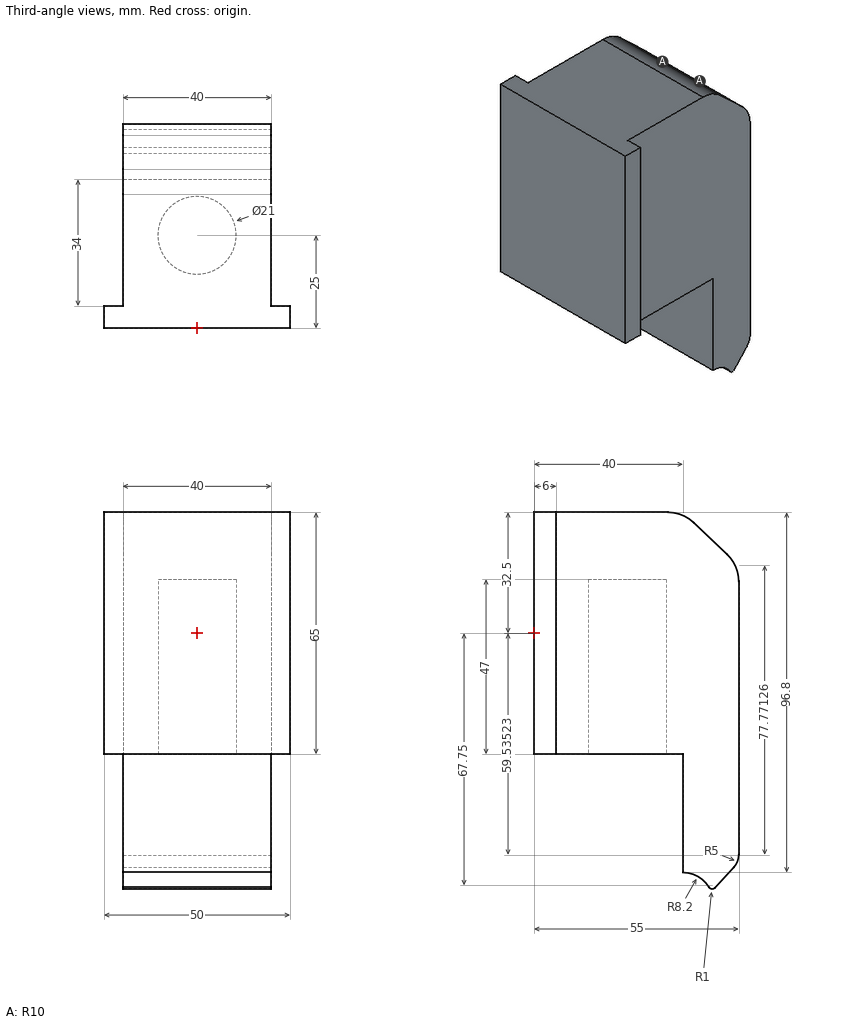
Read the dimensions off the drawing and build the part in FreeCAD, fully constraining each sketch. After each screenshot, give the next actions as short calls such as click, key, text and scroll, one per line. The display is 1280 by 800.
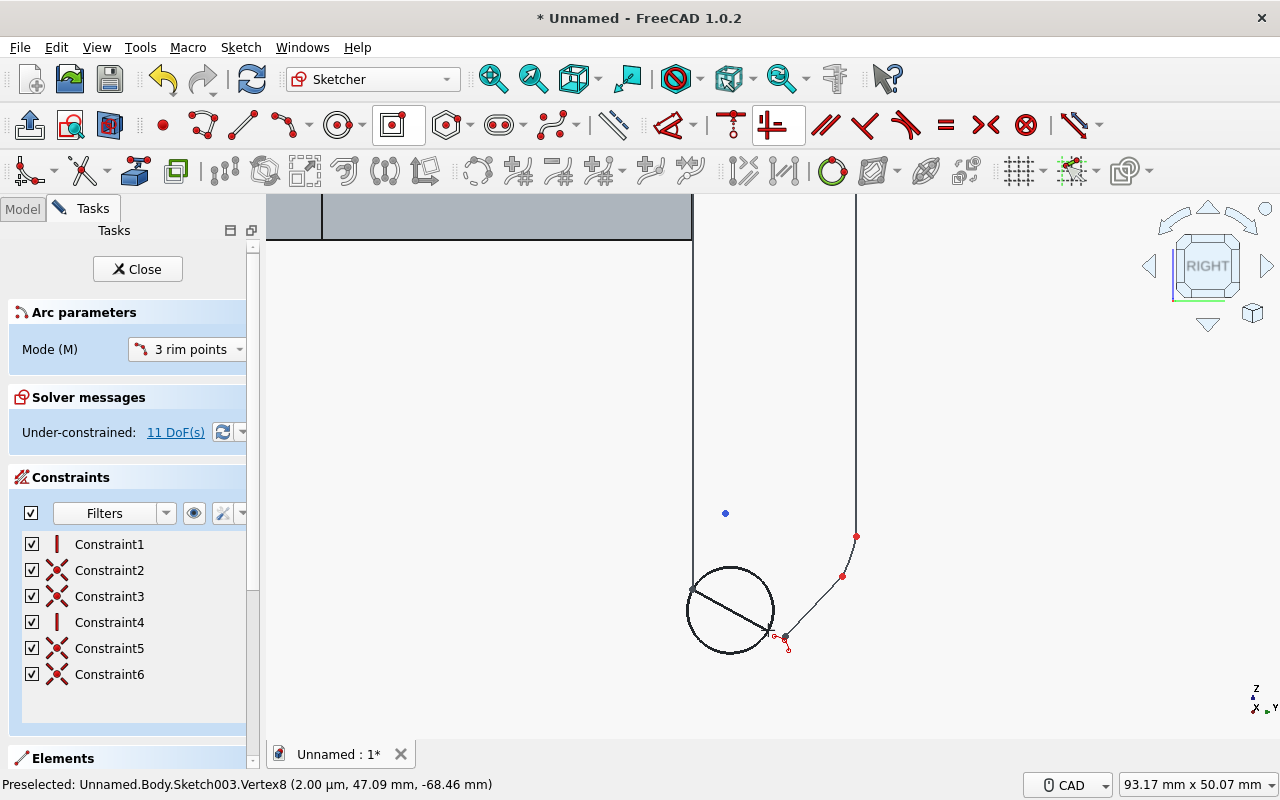
scroll(736, 598, up, 2)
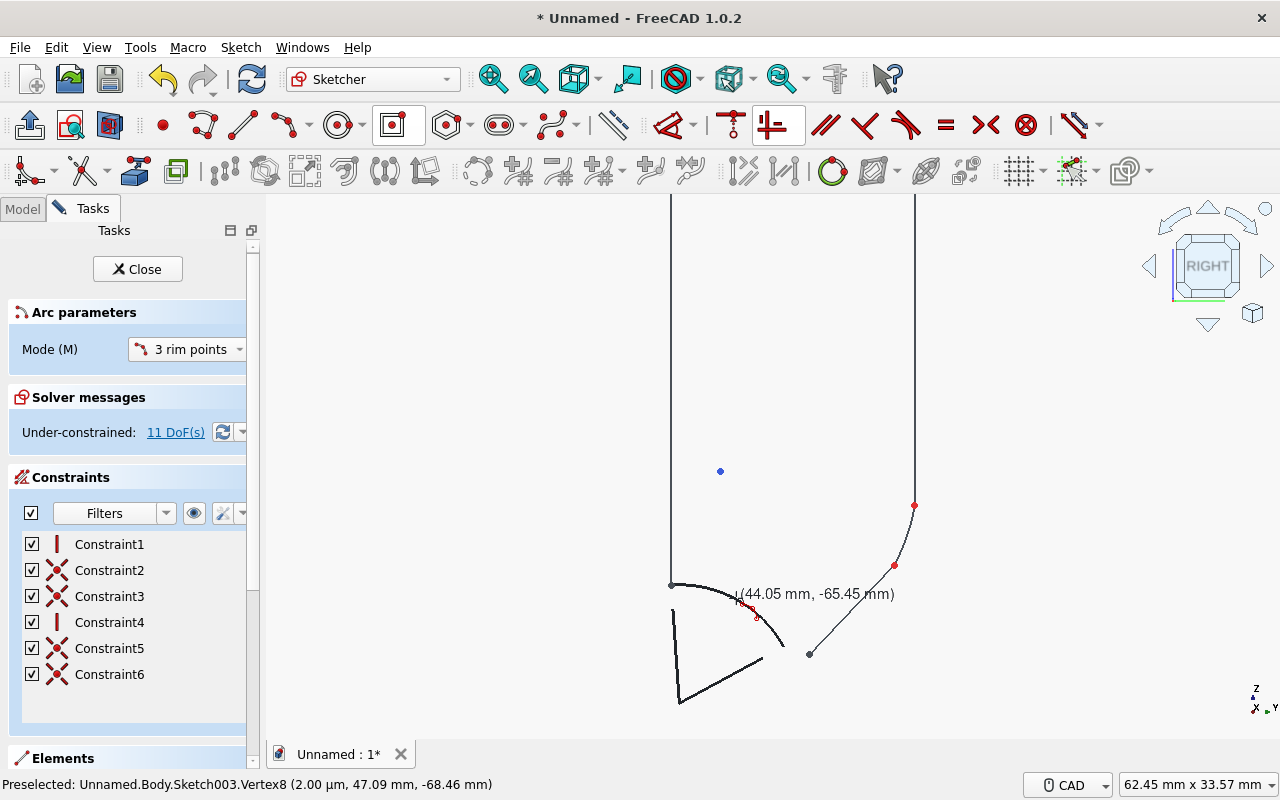
click(735, 598)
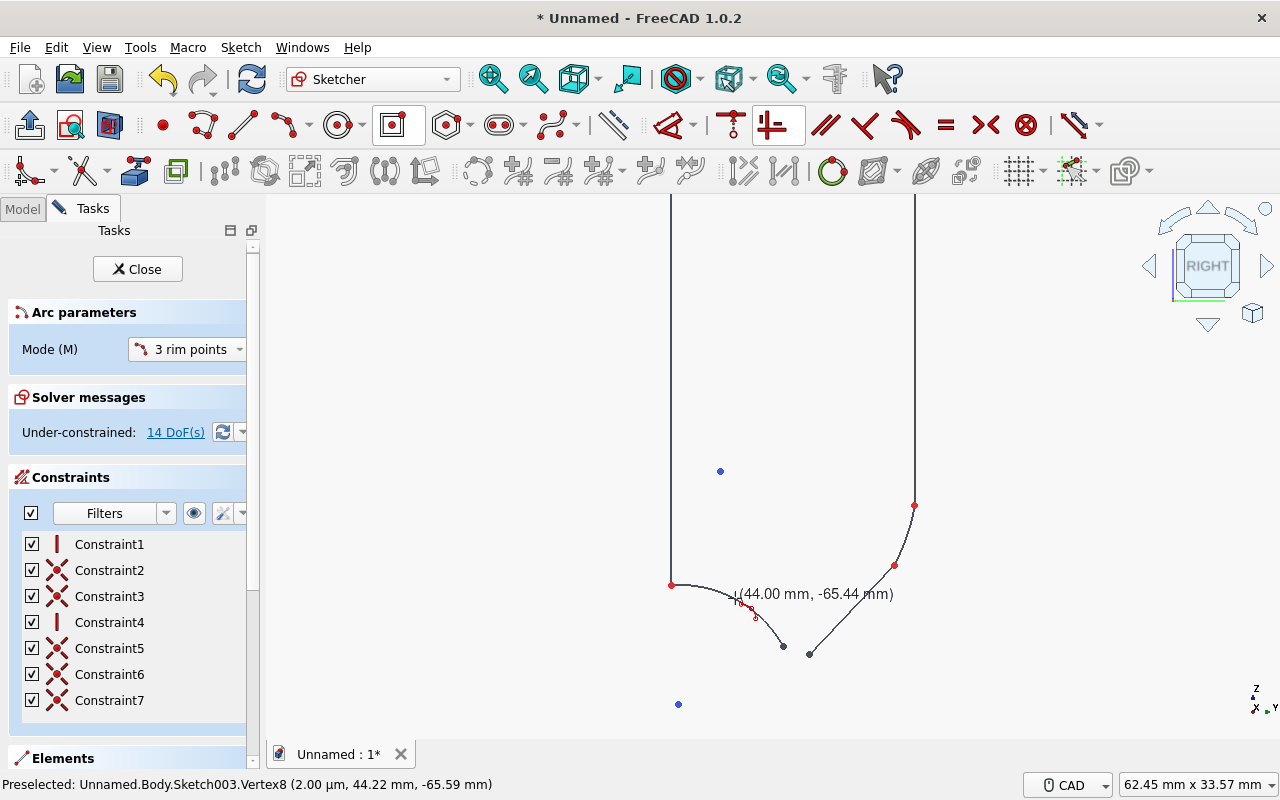
click(784, 647)
click(810, 654)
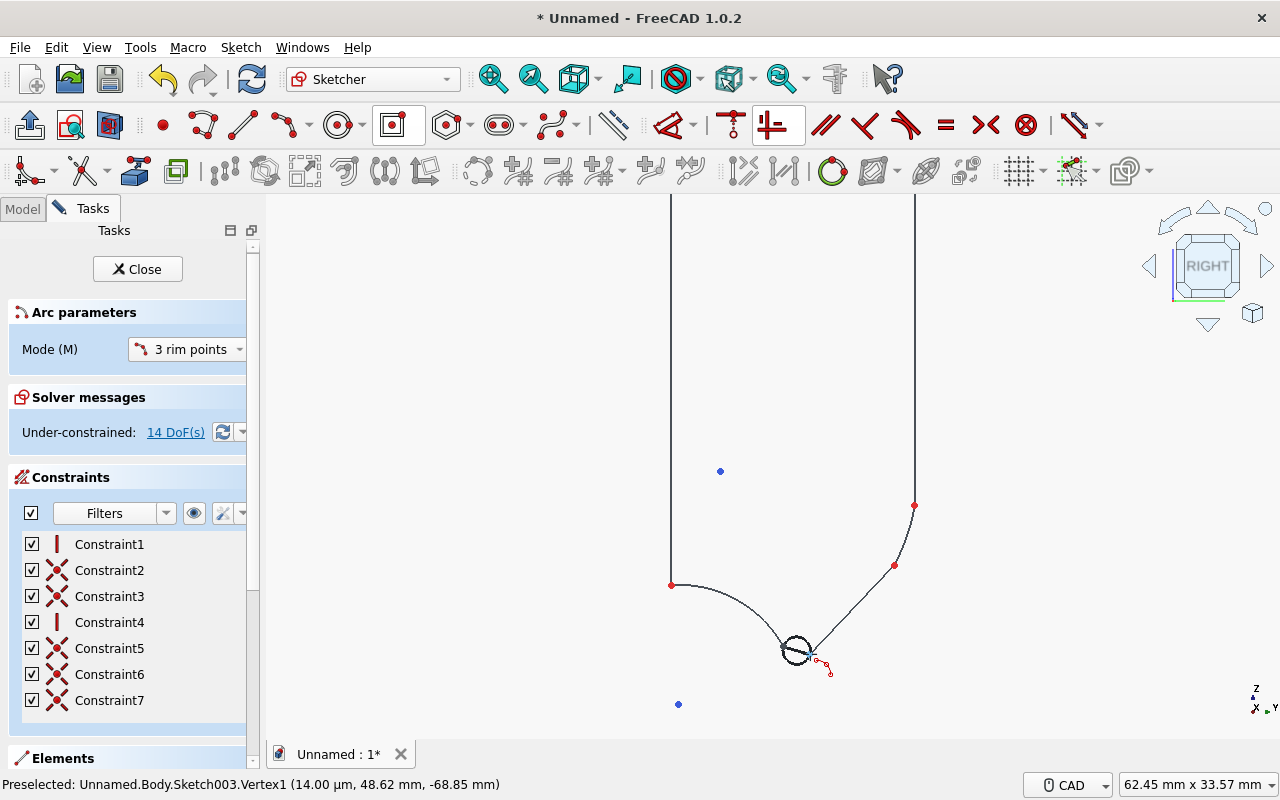
scroll(796, 653, up, 5)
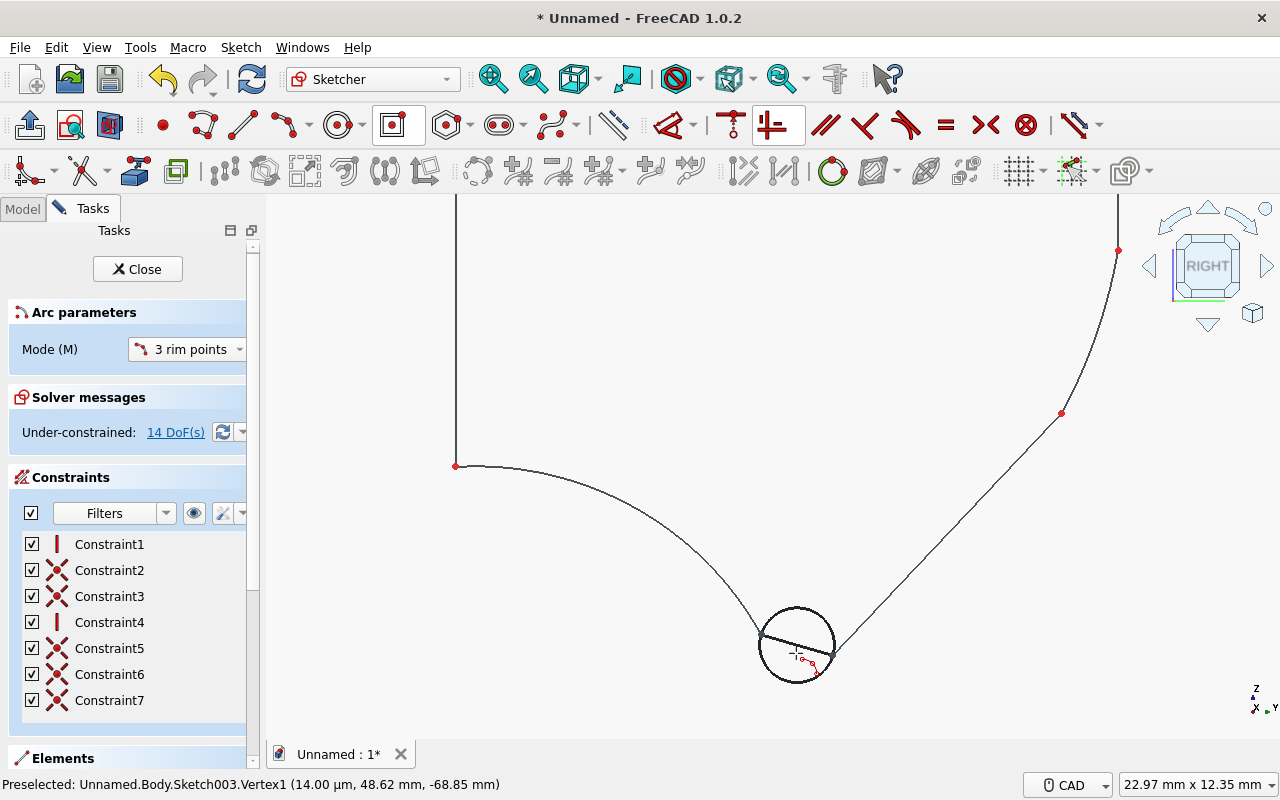
click(796, 651)
key(Escape)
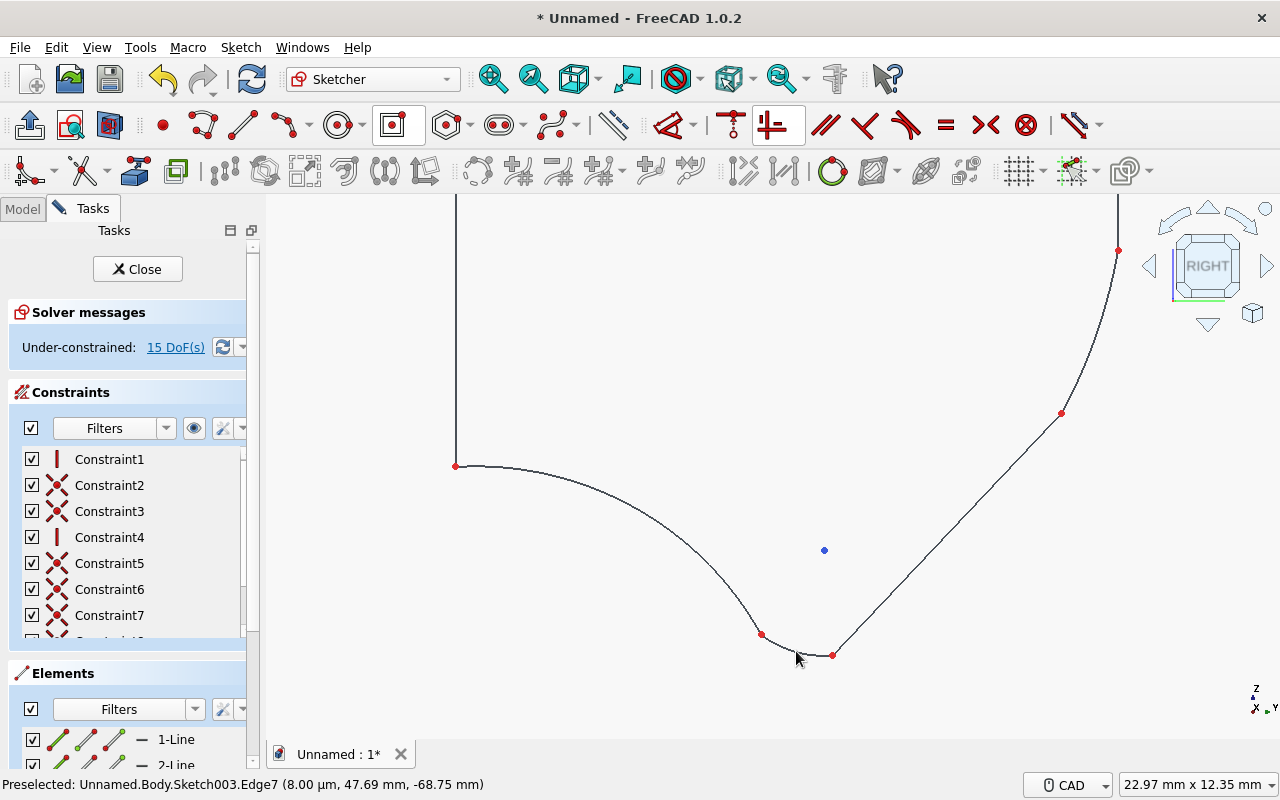
scroll(769, 631, down, 13)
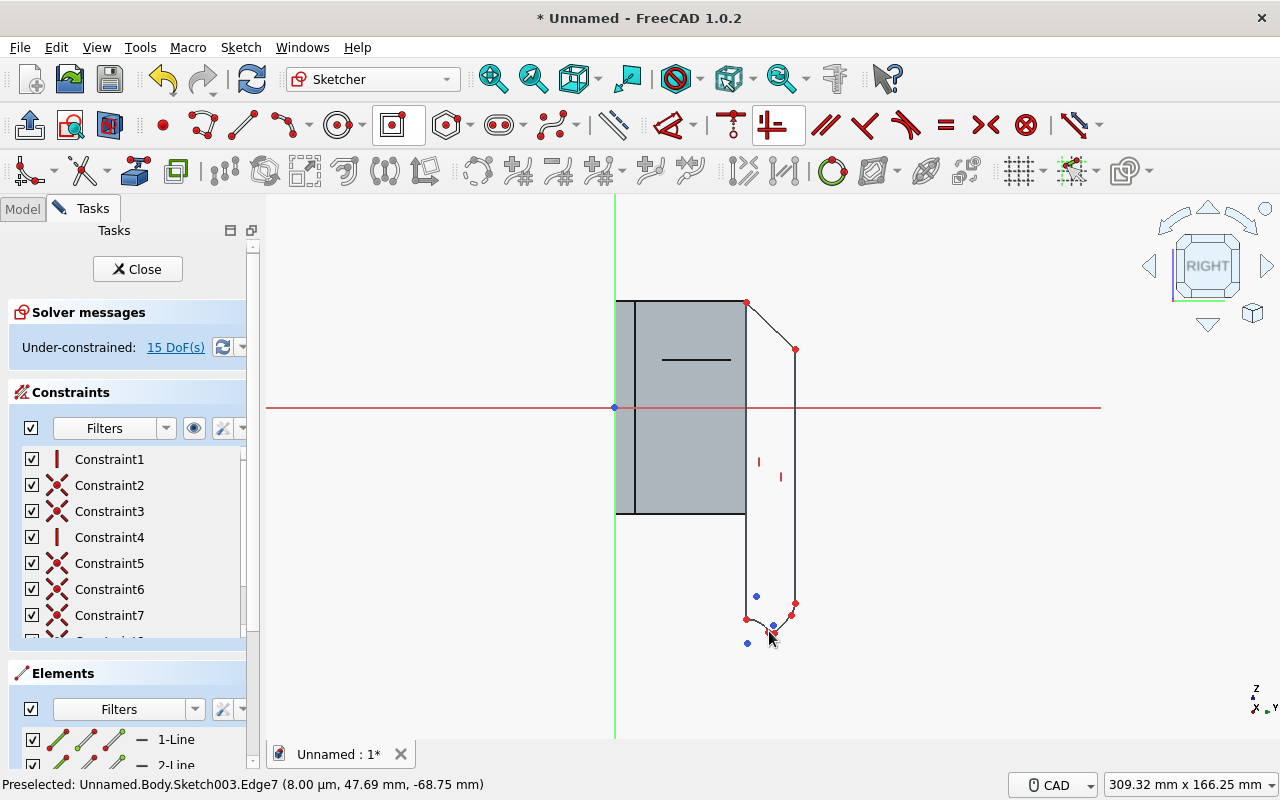
scroll(779, 628, up, 4)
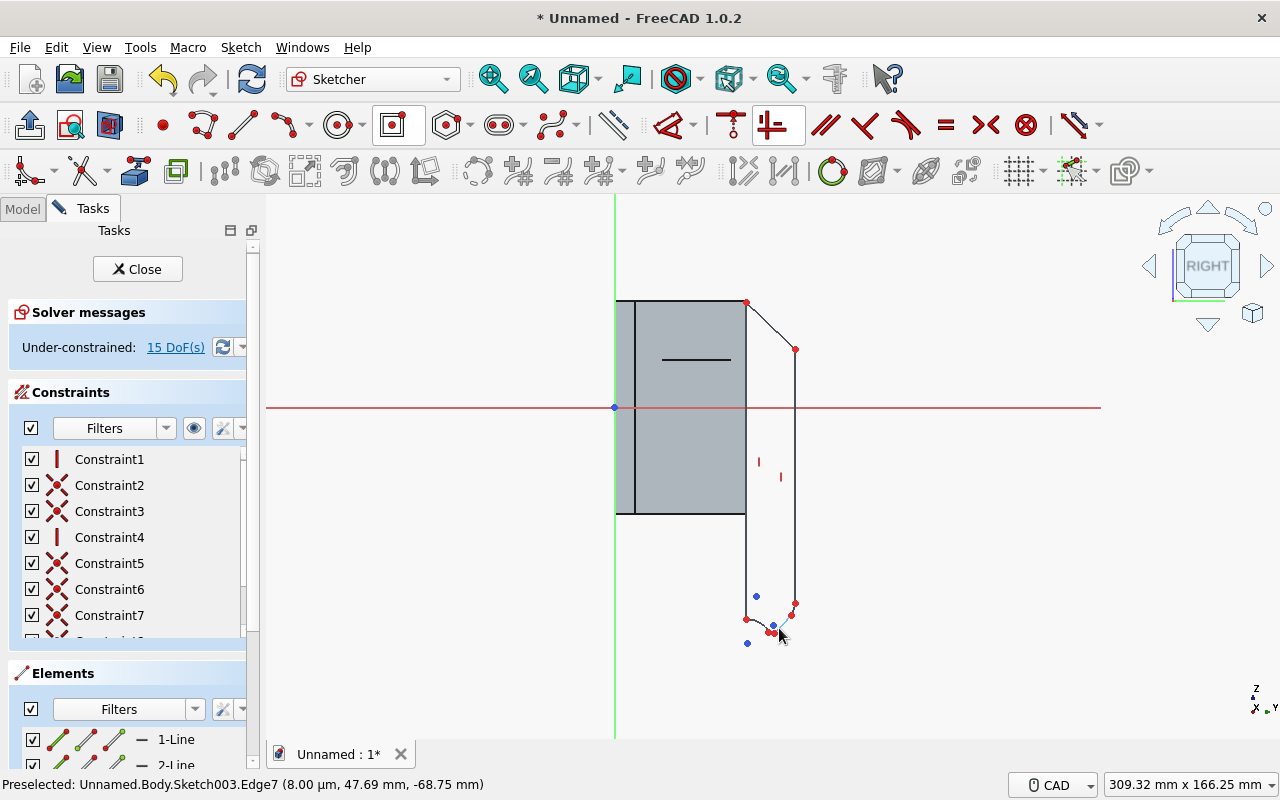
click(779, 627)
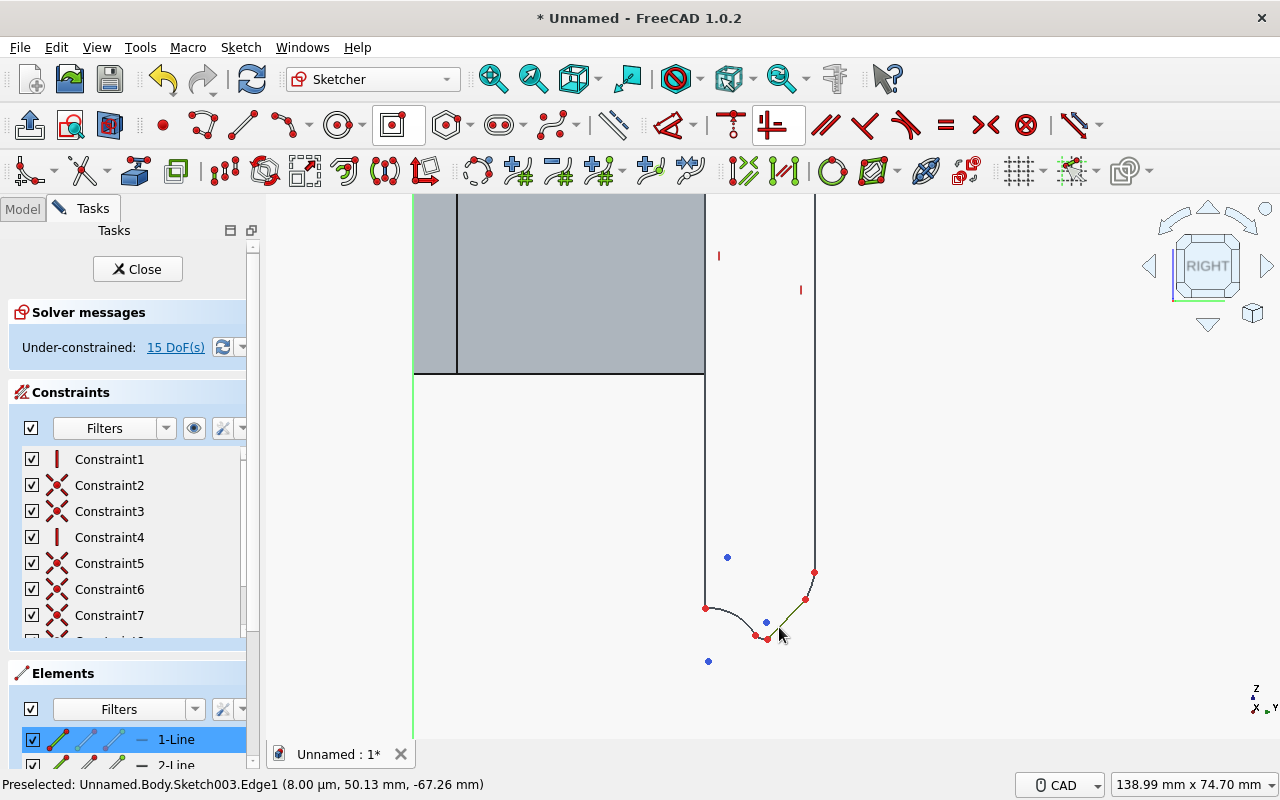
click(811, 586)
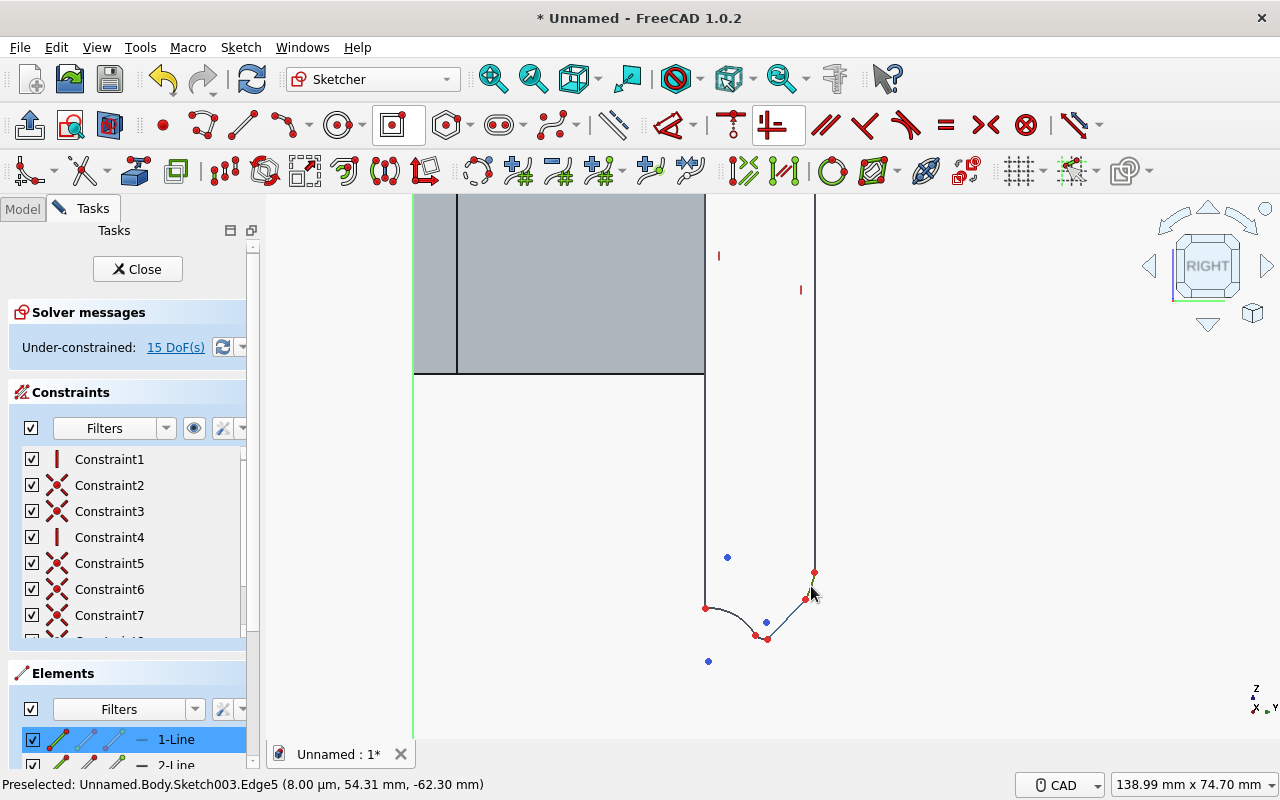
click(906, 126)